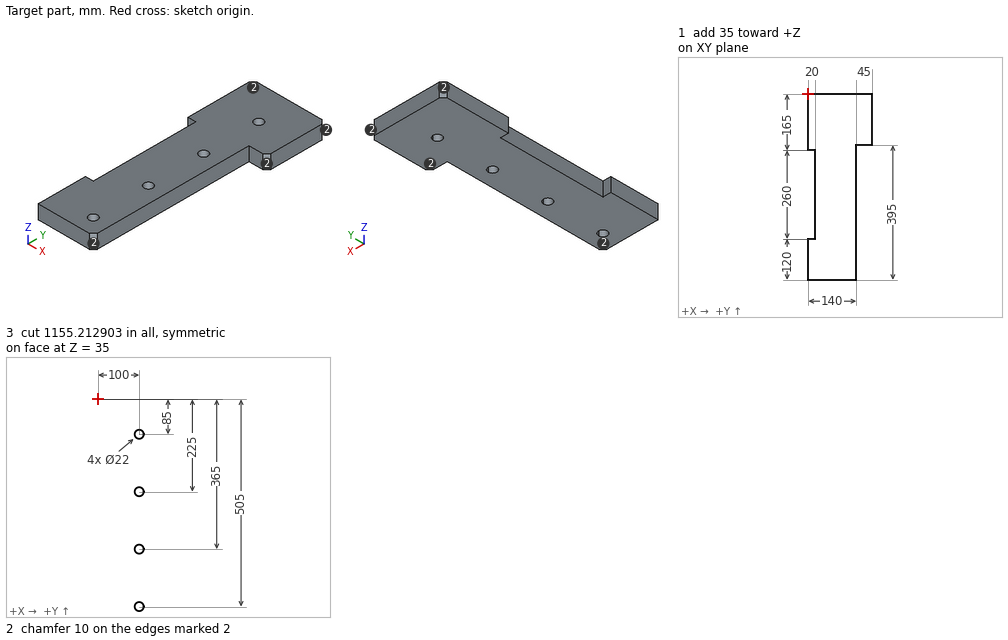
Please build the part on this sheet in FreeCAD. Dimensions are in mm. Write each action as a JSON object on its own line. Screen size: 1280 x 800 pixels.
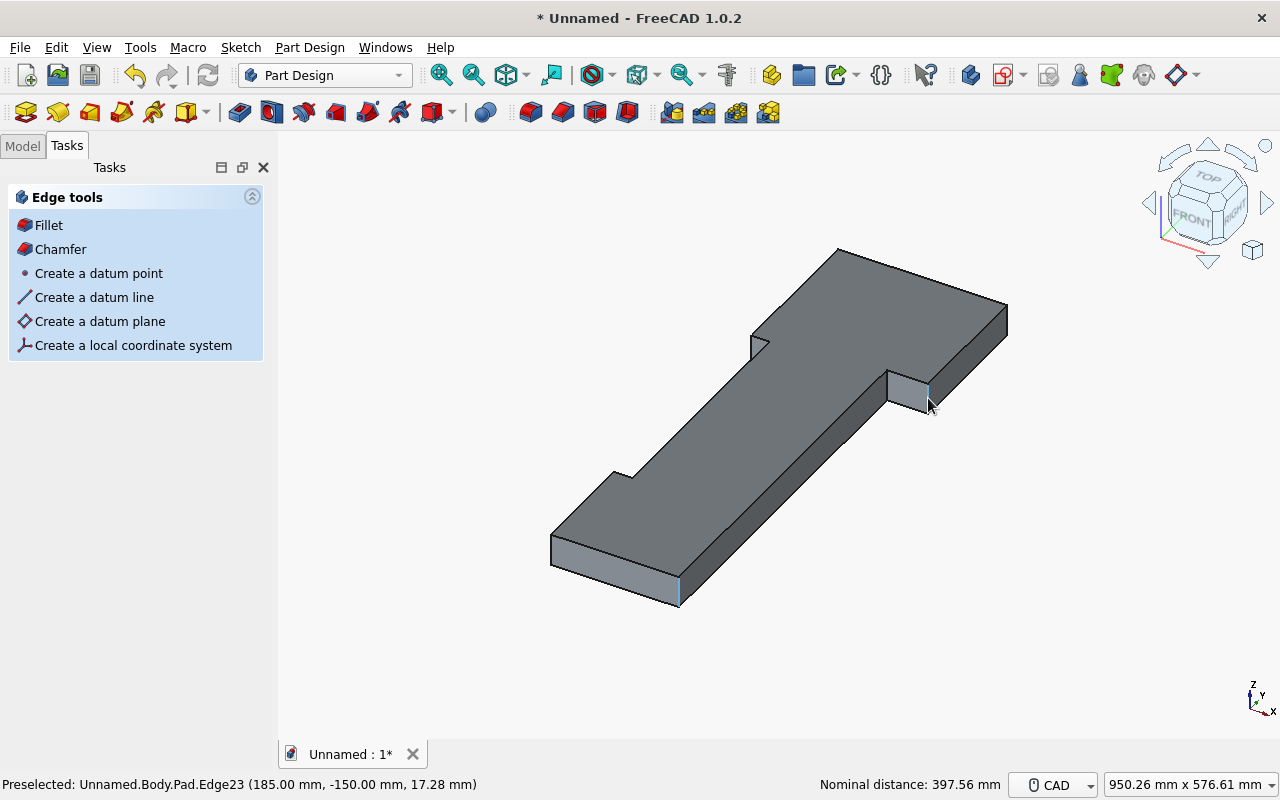
{"action": "key", "text": "0"}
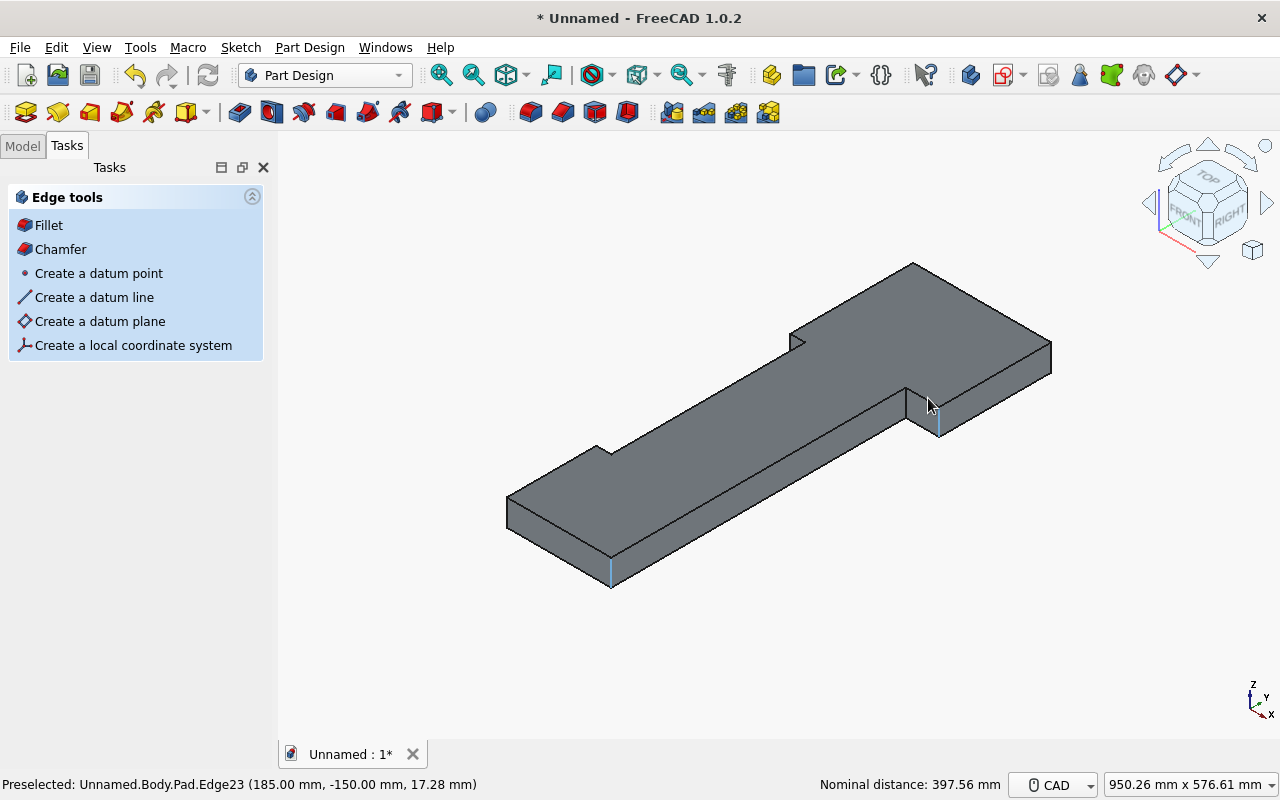
{"action": "key", "text": "2"}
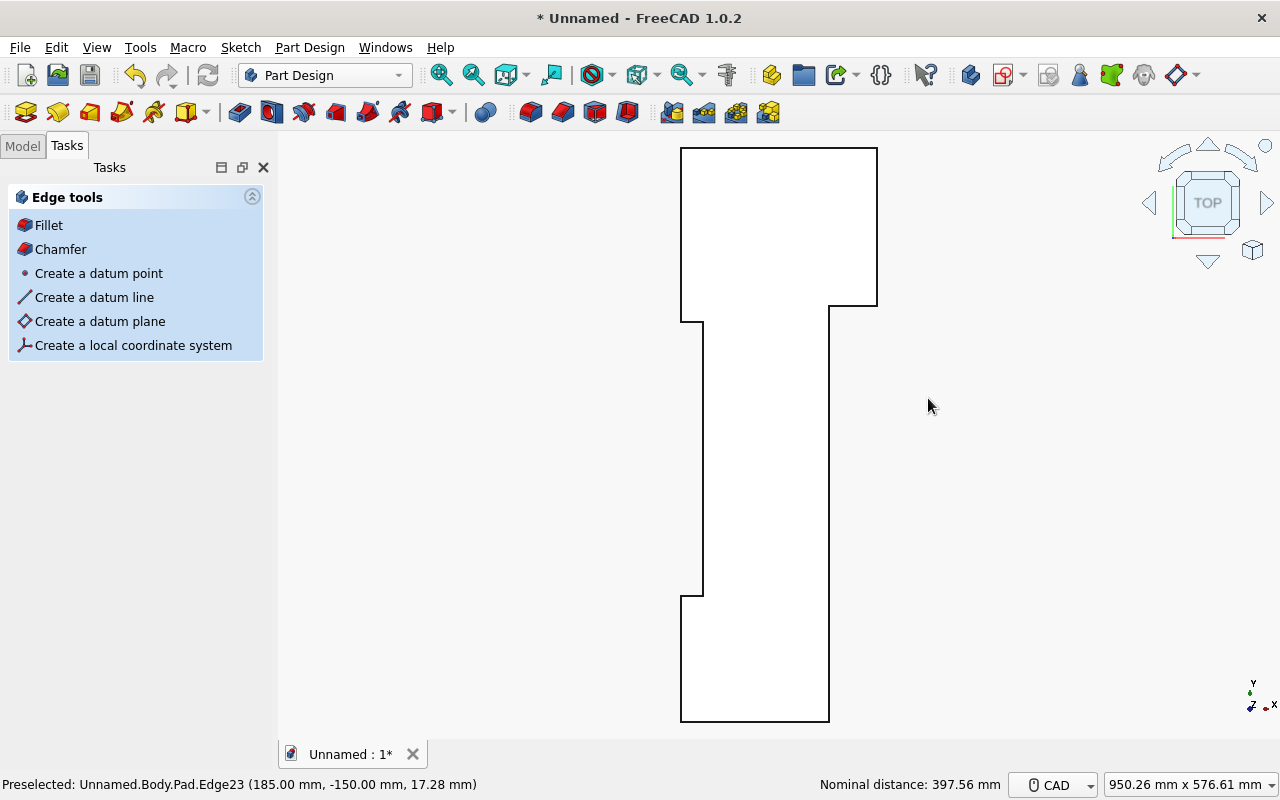
{"action": "key", "text": "1"}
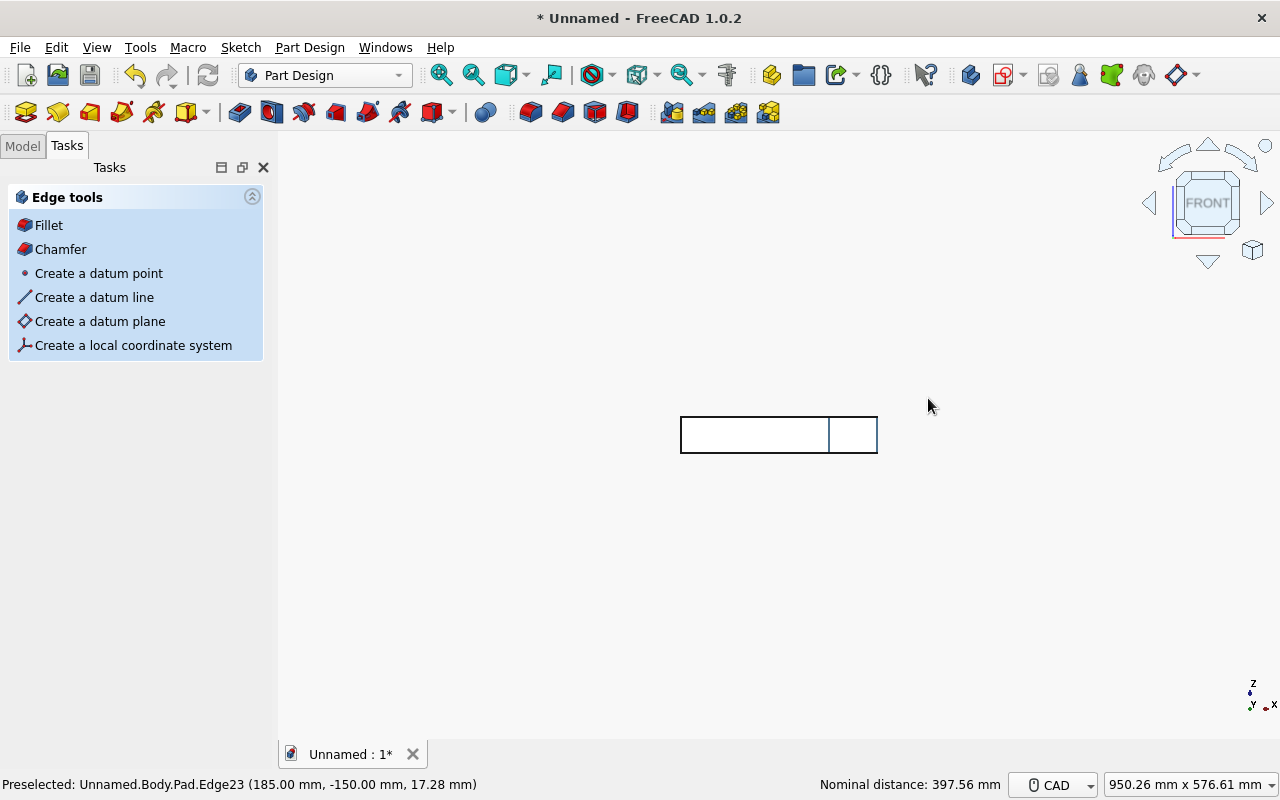
{"action": "left_click", "coordinate": [442, 76]}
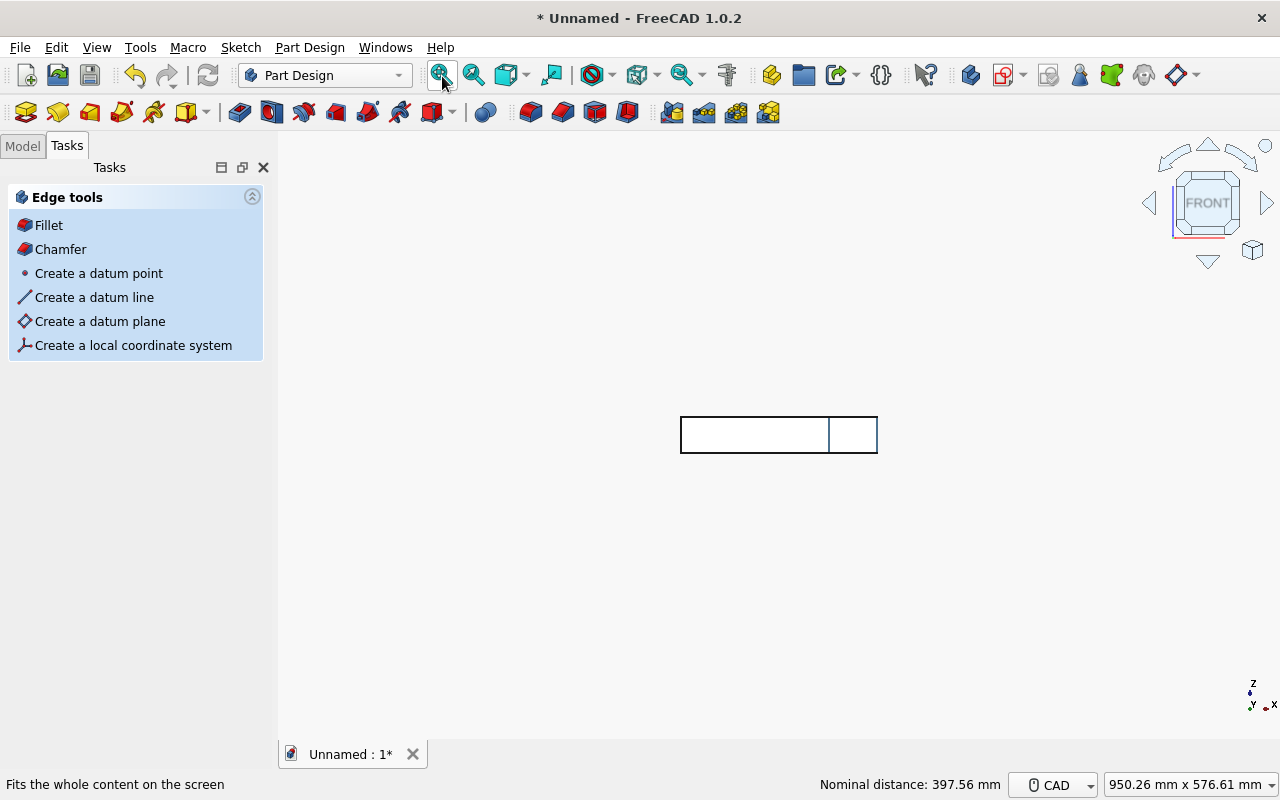
{"action": "key", "text": "3"}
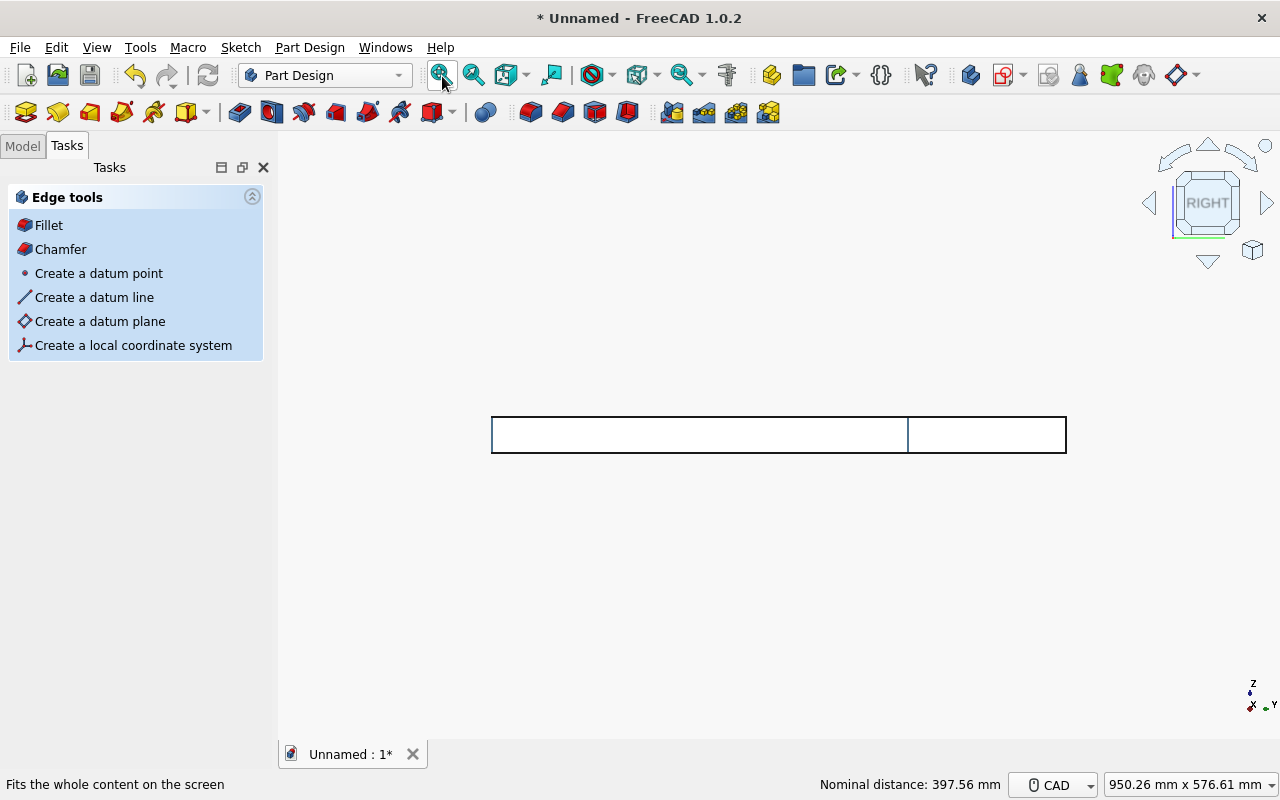
{"action": "left_click", "coordinate": [1066, 434], "text": "ctrl"}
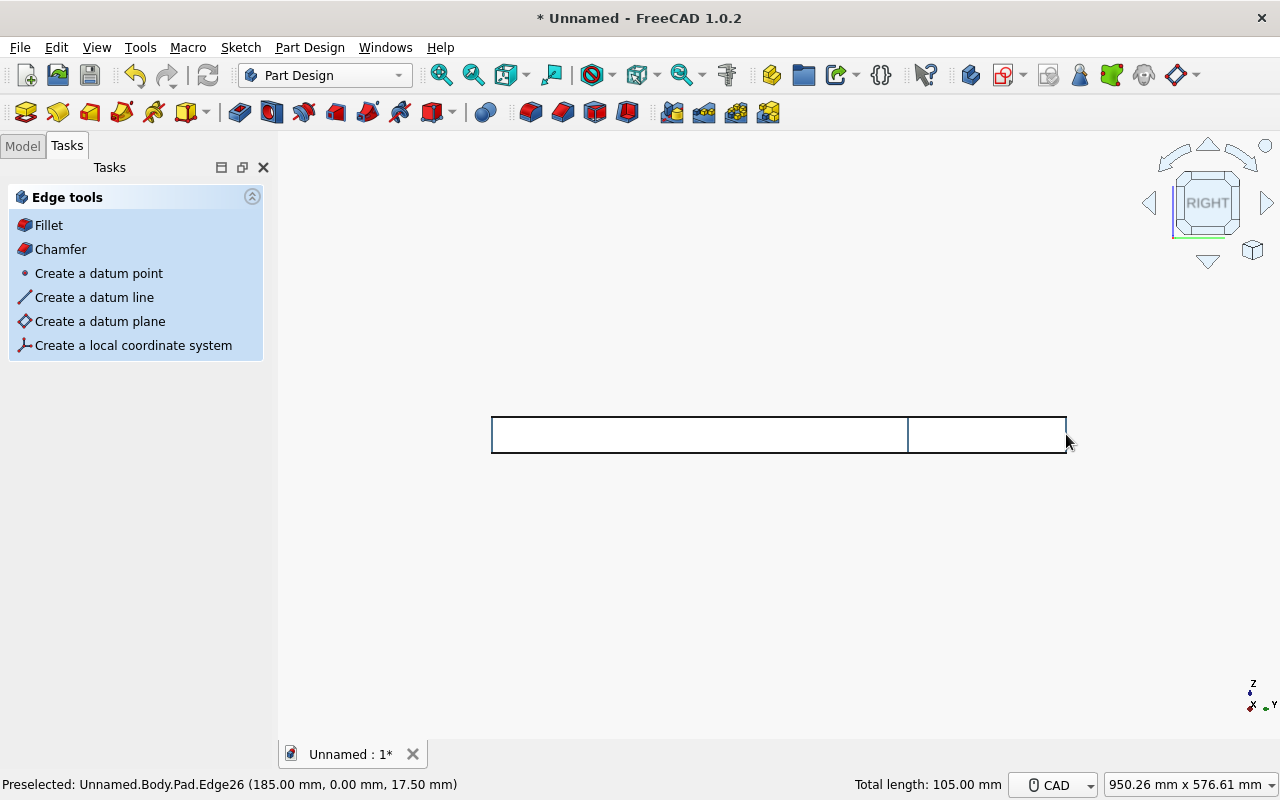
{"action": "key", "text": "5"}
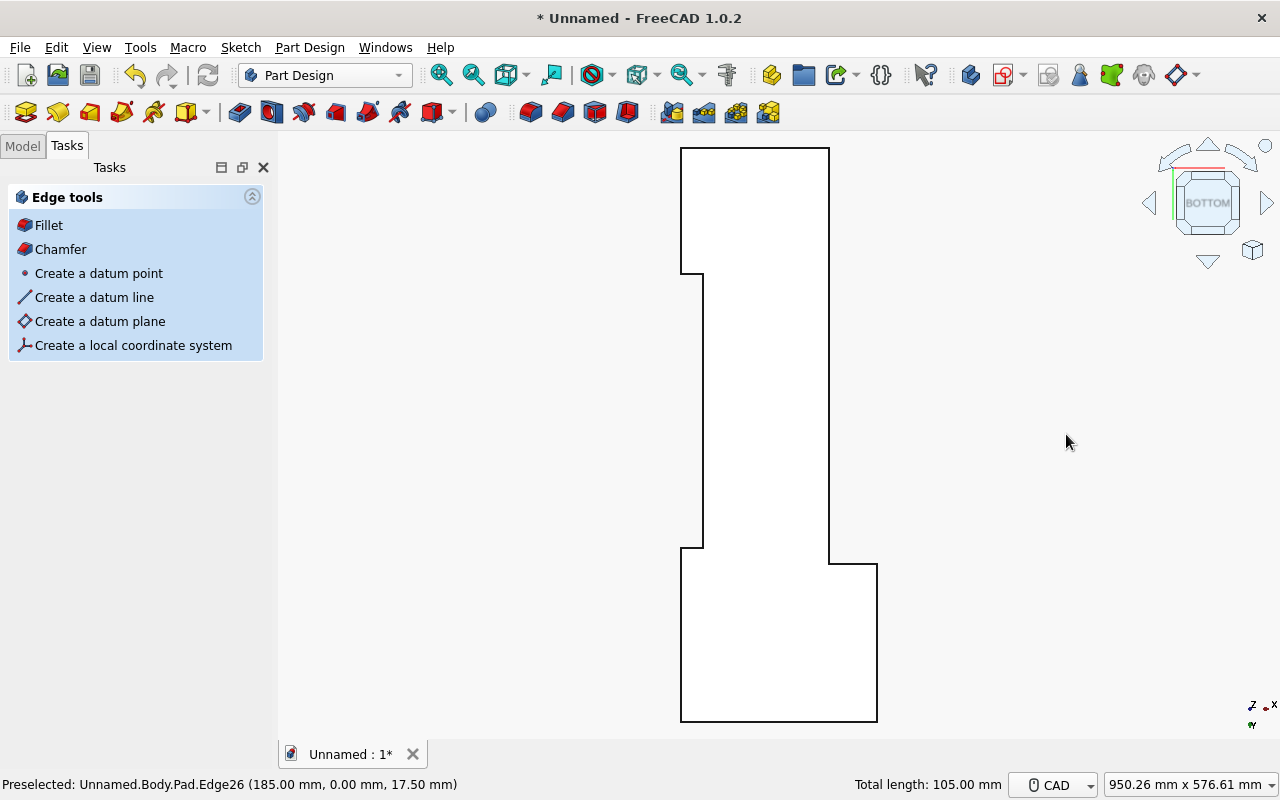
{"action": "key", "text": "4"}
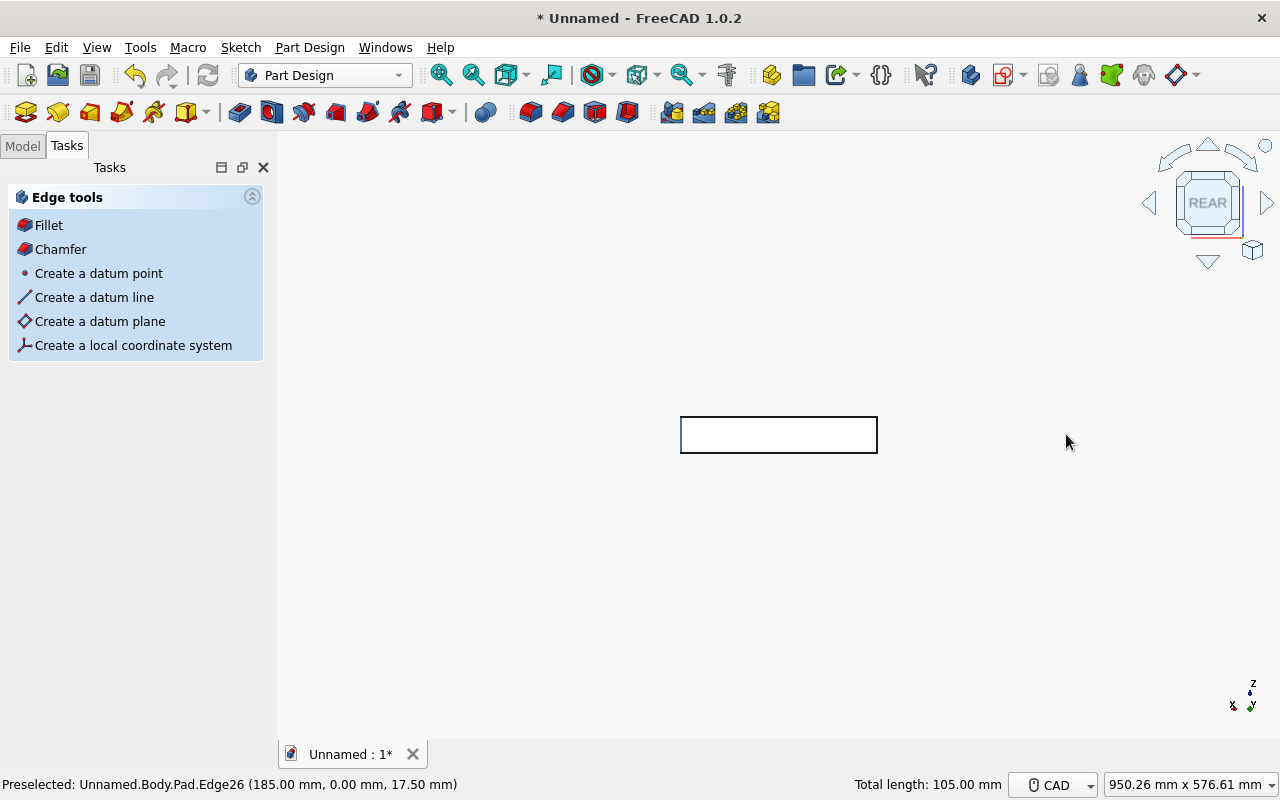
{"action": "left_click", "coordinate": [442, 76]}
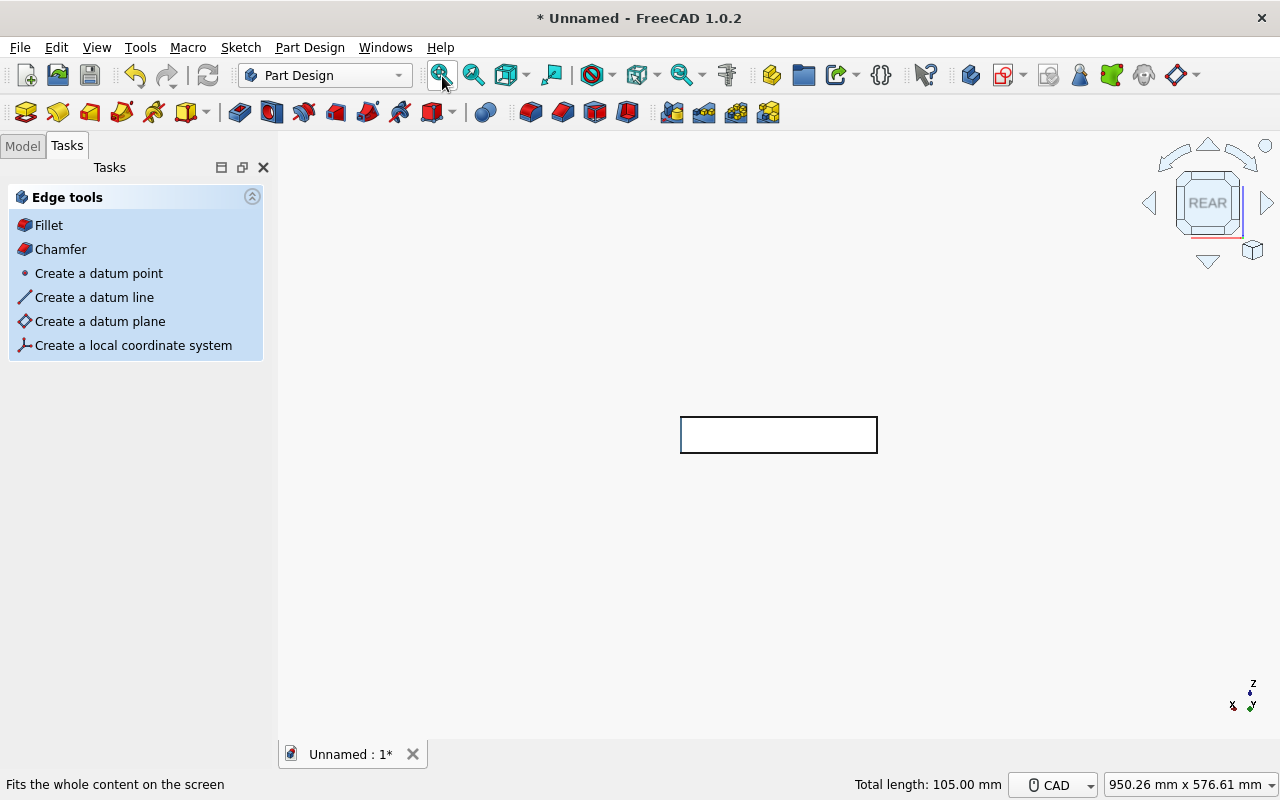
{"action": "left_click", "coordinate": [877, 434], "text": "ctrl"}